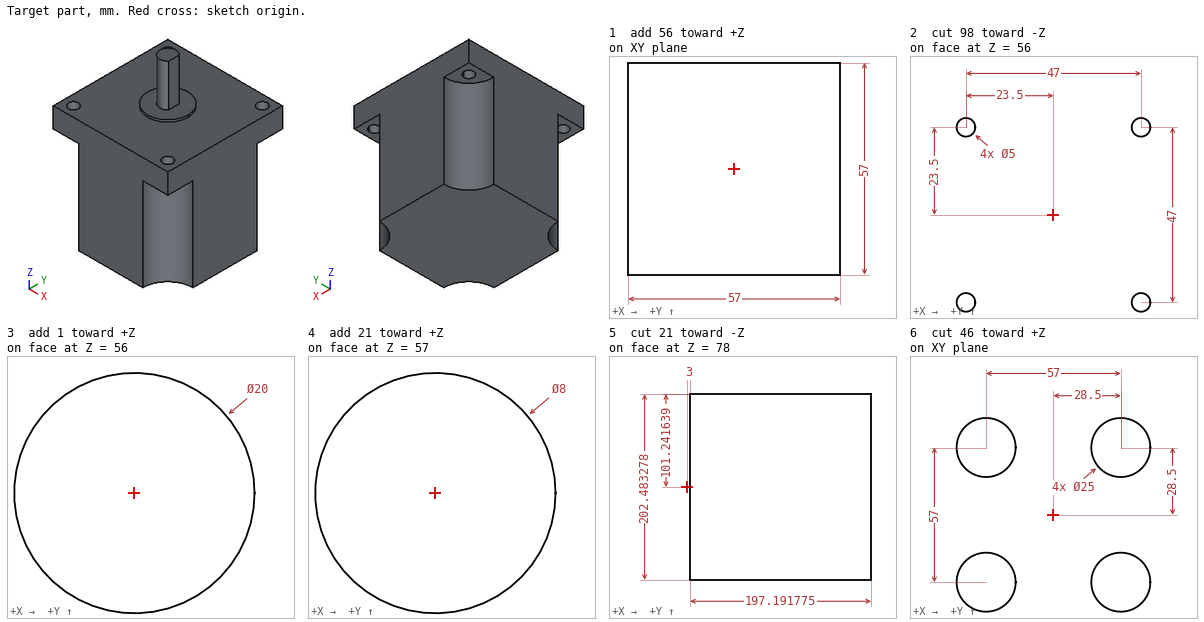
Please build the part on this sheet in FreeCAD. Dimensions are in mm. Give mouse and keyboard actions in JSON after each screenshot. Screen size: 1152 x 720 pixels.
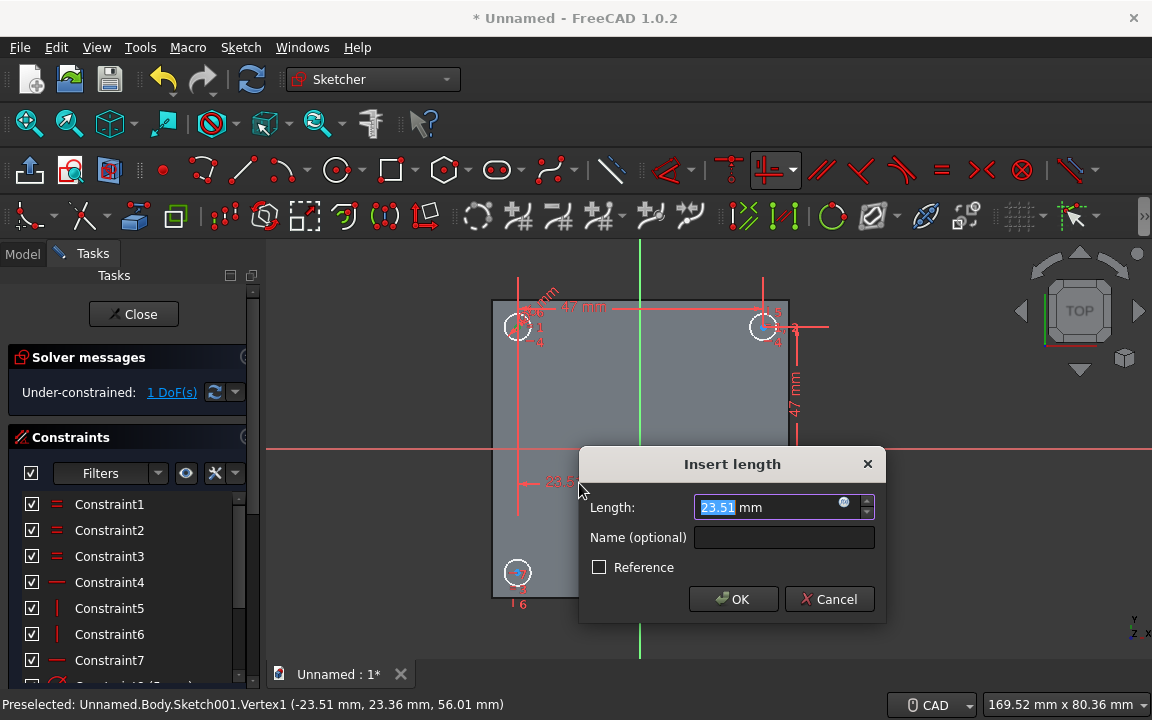
{"action": "type", "text": "23.5"}
{"action": "key", "text": "Return"}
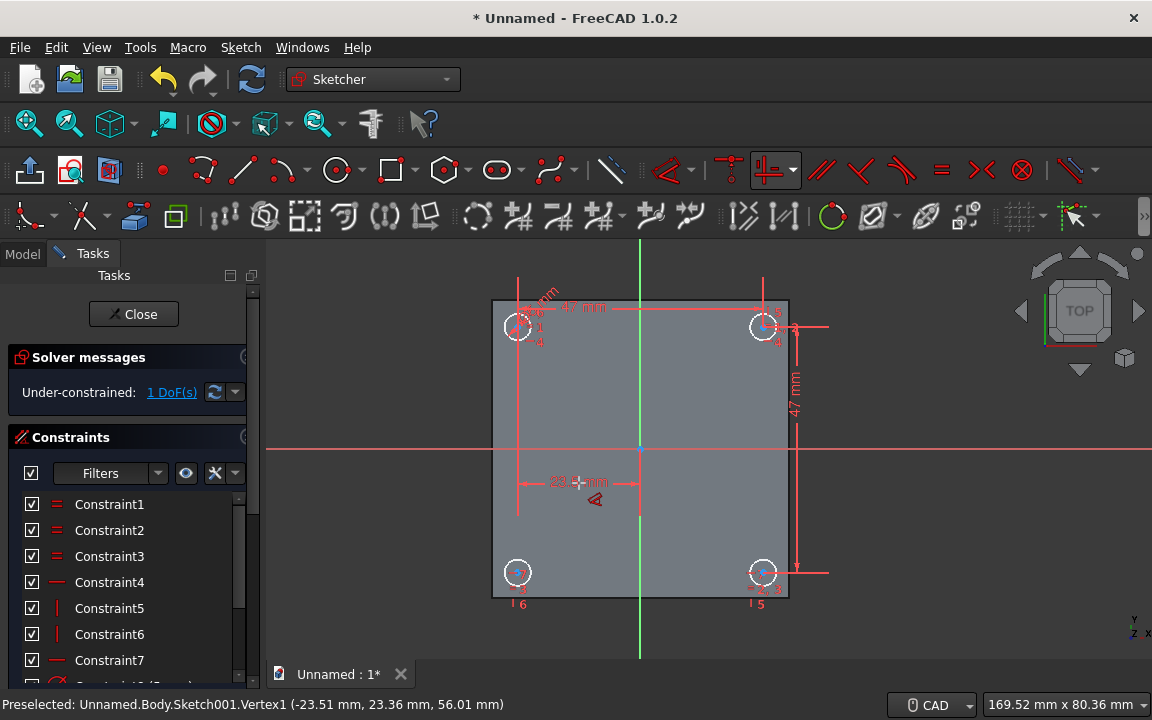
{"action": "left_click", "coordinate": [518, 327]}
{"action": "left_click", "coordinate": [484, 388]}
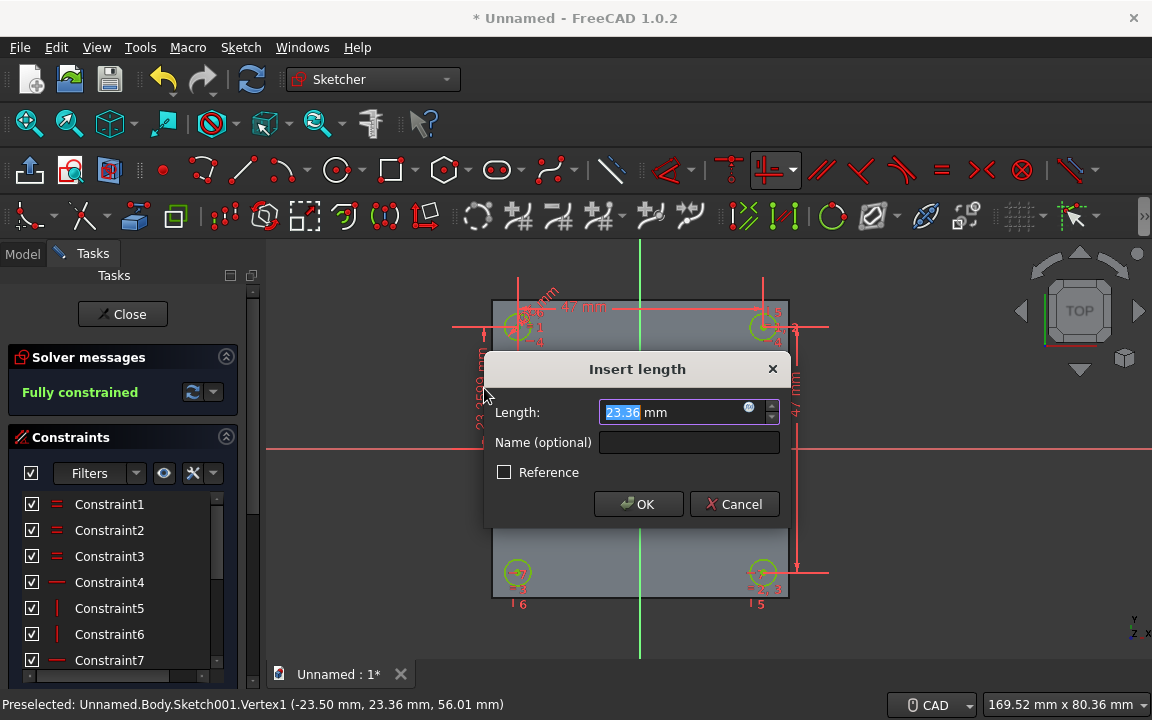
{"action": "type", "text": "23.5"}
{"action": "key", "text": "Return"}
{"action": "key", "text": "Escape"}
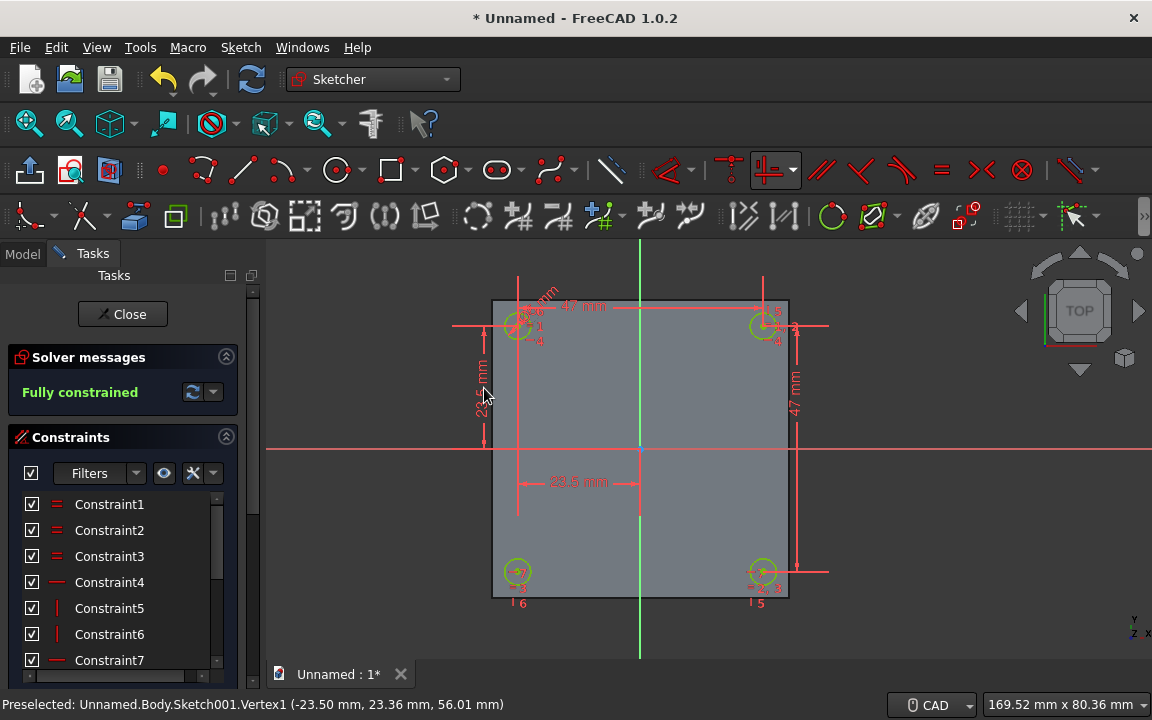
{"action": "left_click", "coordinate": [123, 314]}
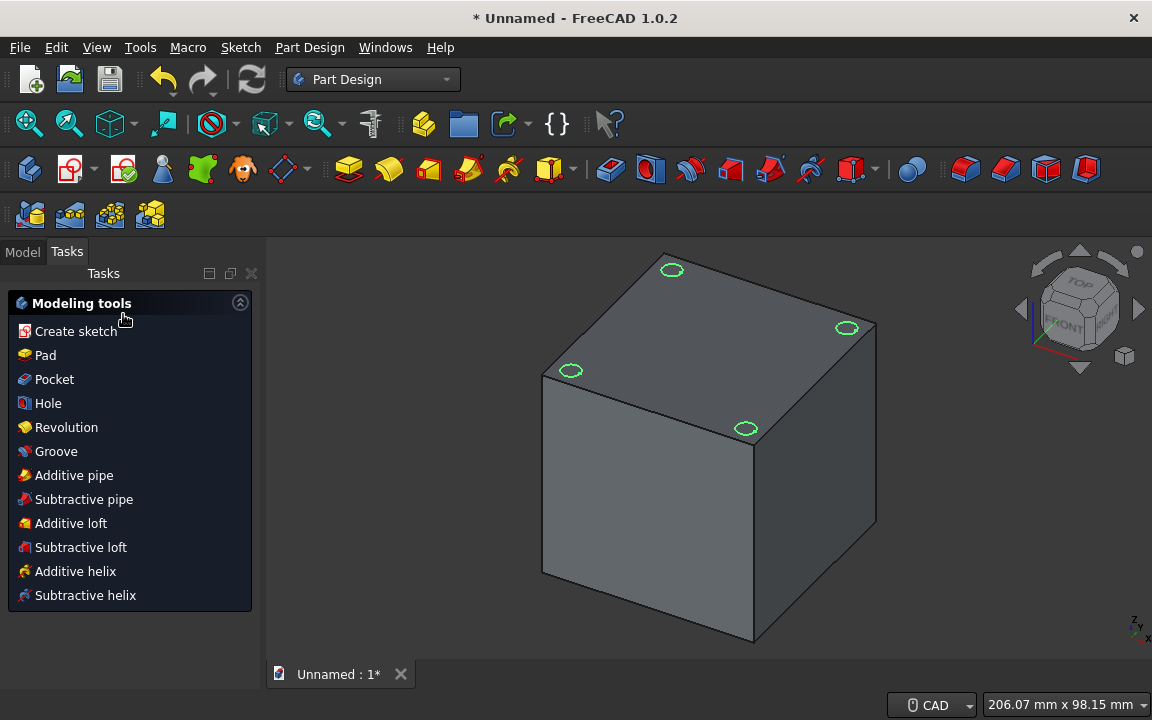
{"action": "left_click", "coordinate": [612, 170]}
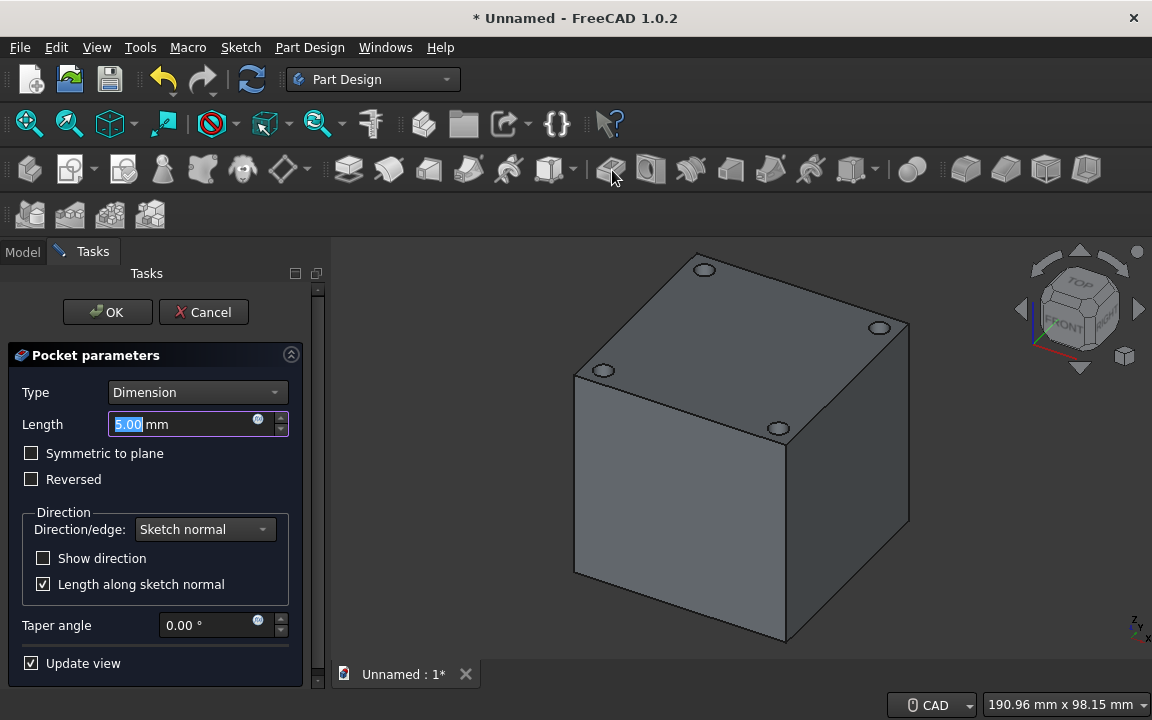
{"action": "type", "text": "98"}
{"action": "key", "text": "Tab"}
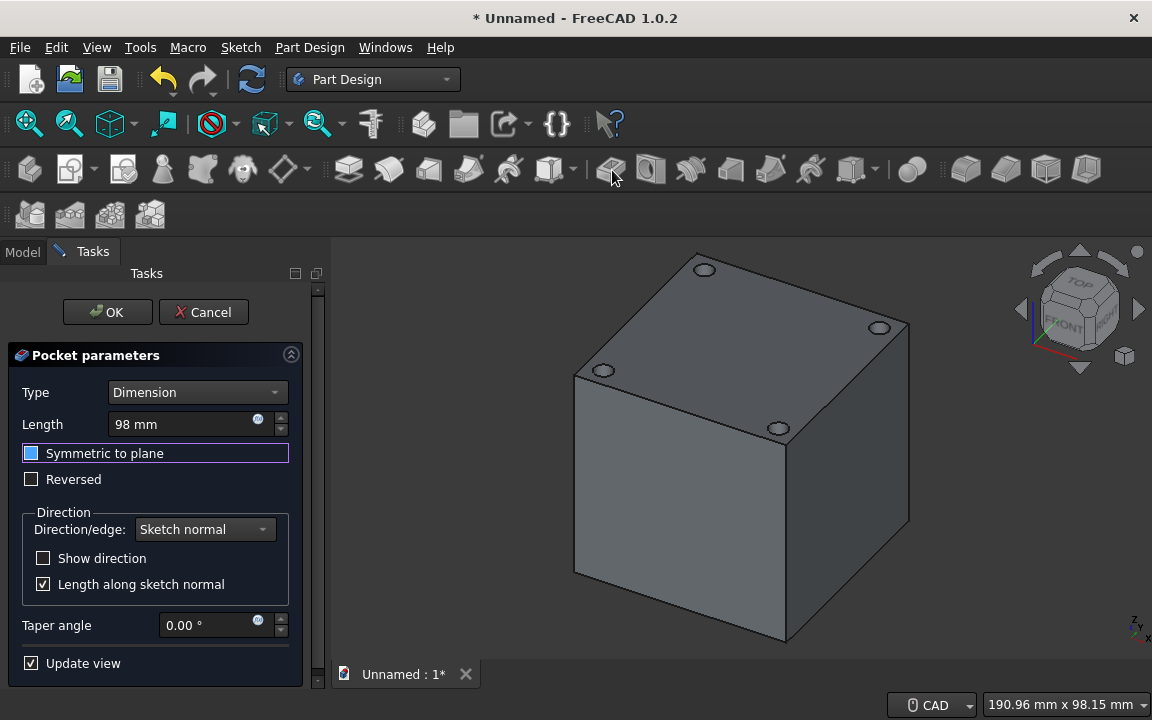
{"action": "left_click", "coordinate": [108, 312]}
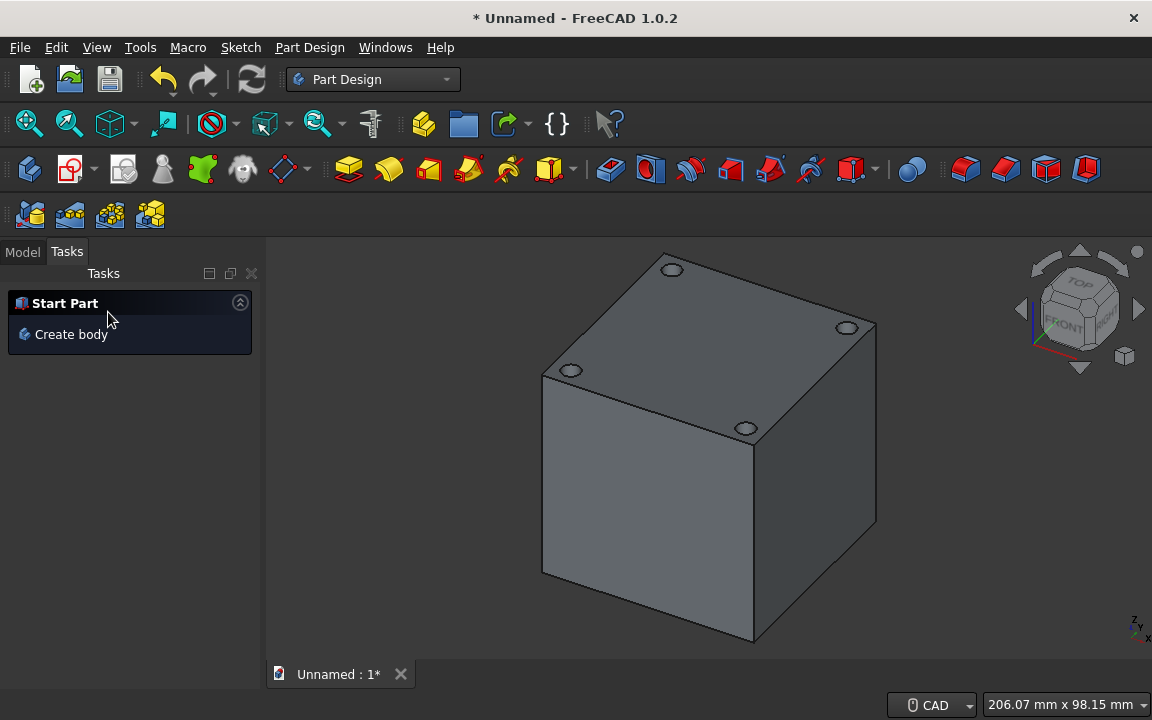
{"action": "left_click", "coordinate": [709, 348]}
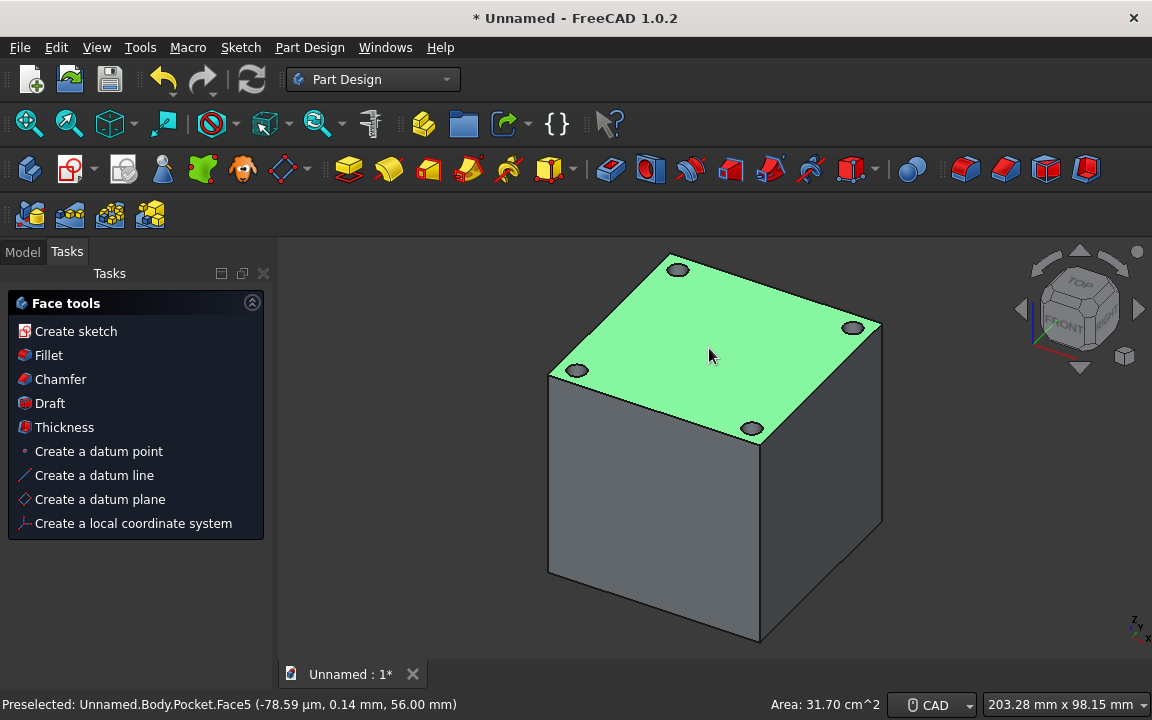
{"action": "left_click", "coordinate": [70, 170]}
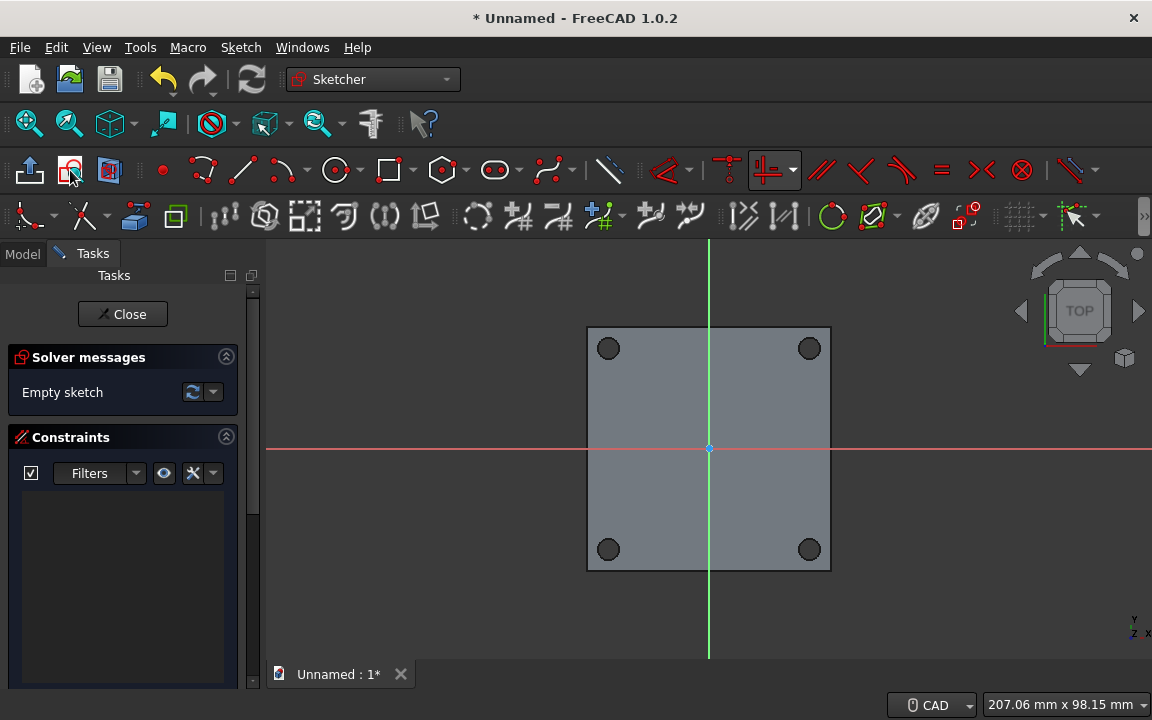
{"action": "scroll", "coordinate": [749, 449], "scroll_direction": "up", "scroll_amount": 5}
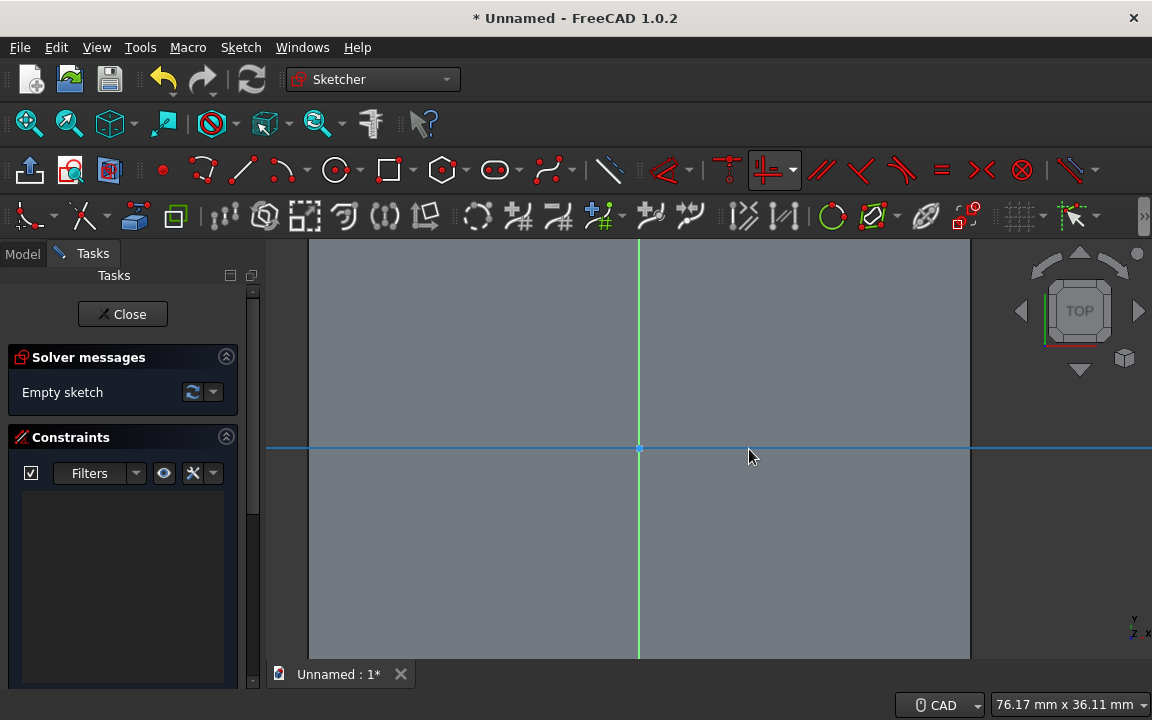
{"action": "left_click", "coordinate": [336, 170]}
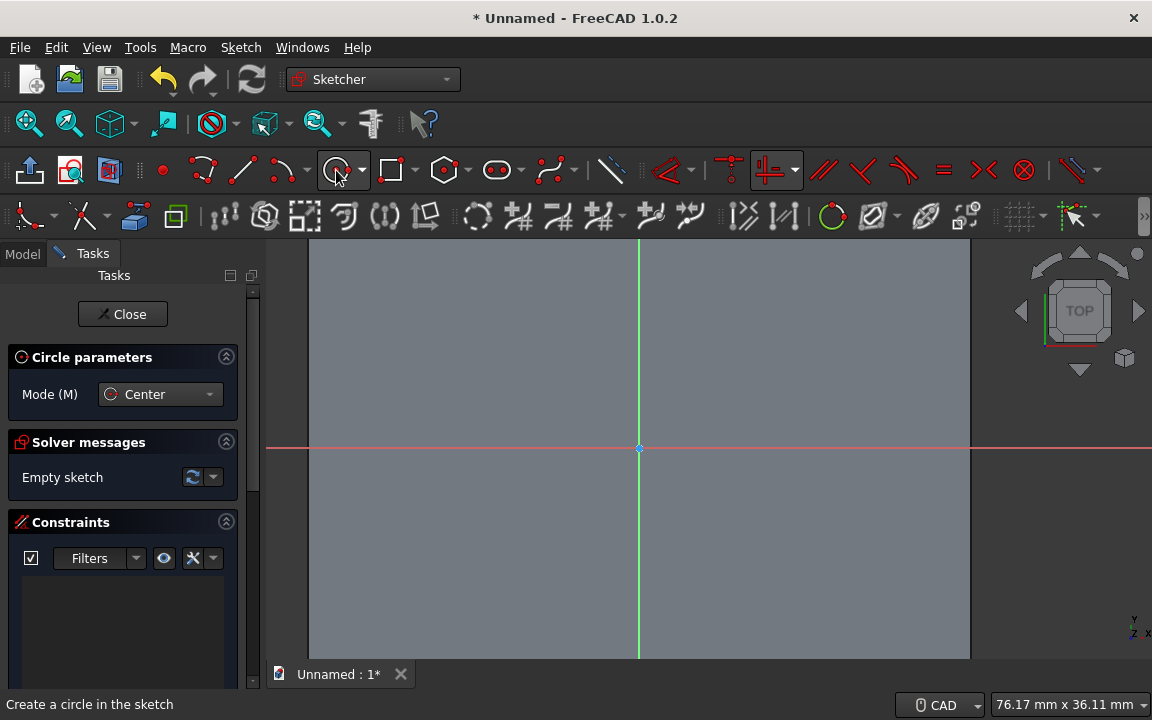
{"action": "left_click", "coordinate": [639, 448]}
{"action": "left_click", "coordinate": [722, 366]}
{"action": "key", "text": "Escape"}